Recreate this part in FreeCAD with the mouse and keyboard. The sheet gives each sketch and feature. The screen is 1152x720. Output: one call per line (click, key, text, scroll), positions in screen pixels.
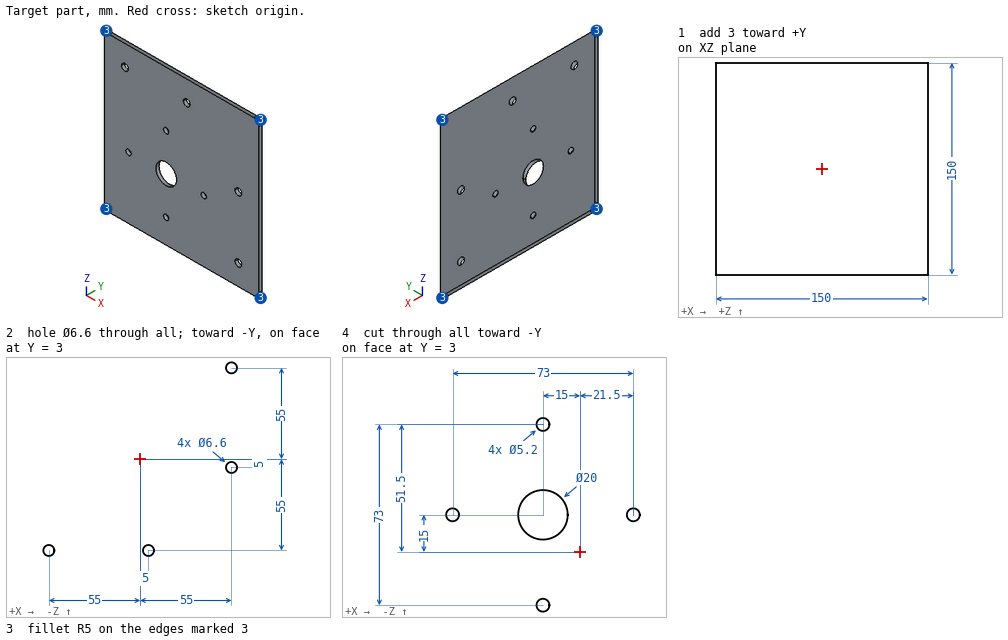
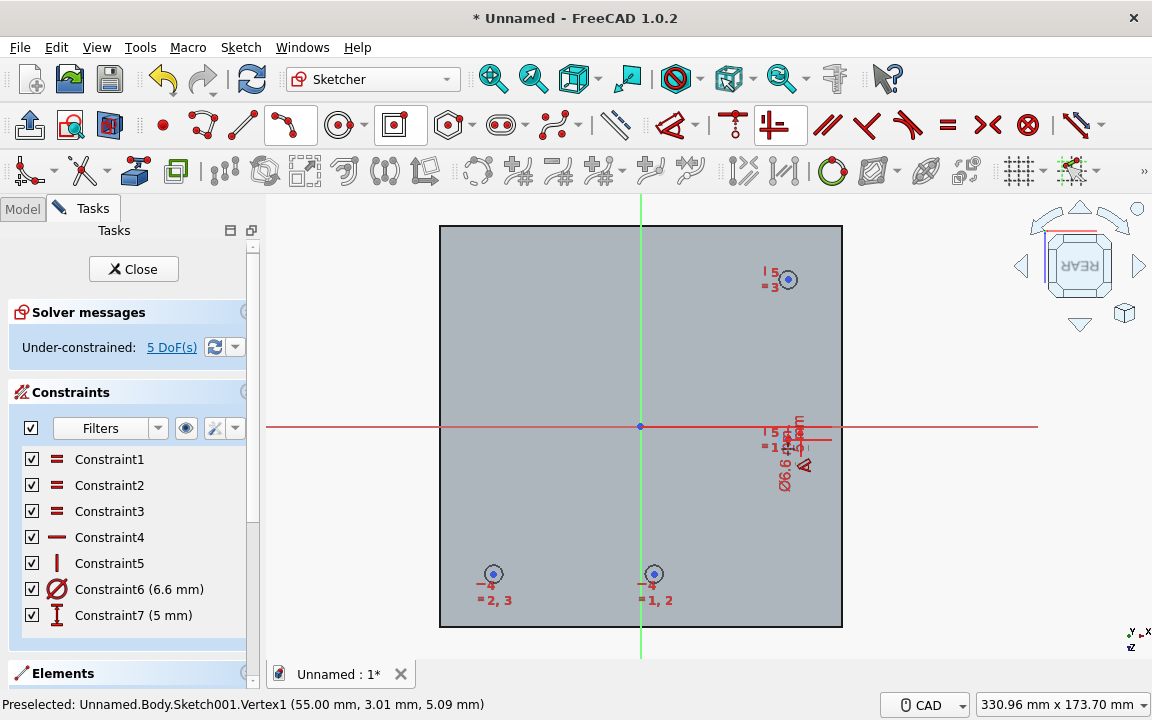
scroll(654, 574, up, 6)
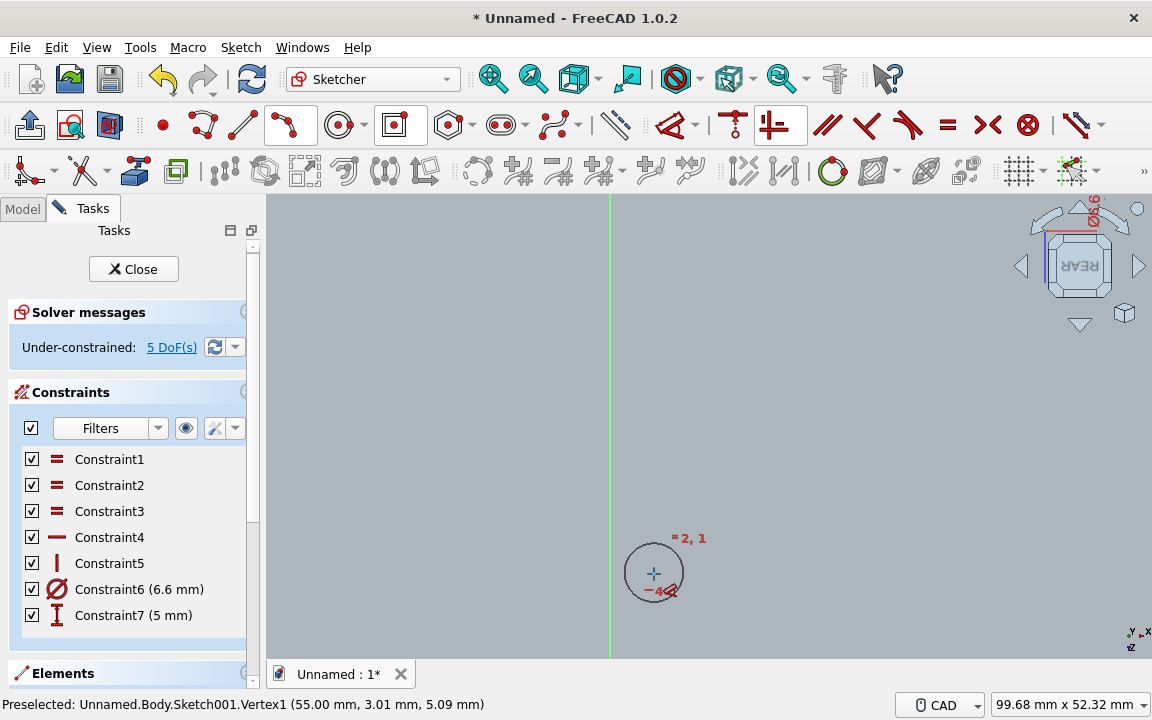
click(654, 573)
click(632, 631)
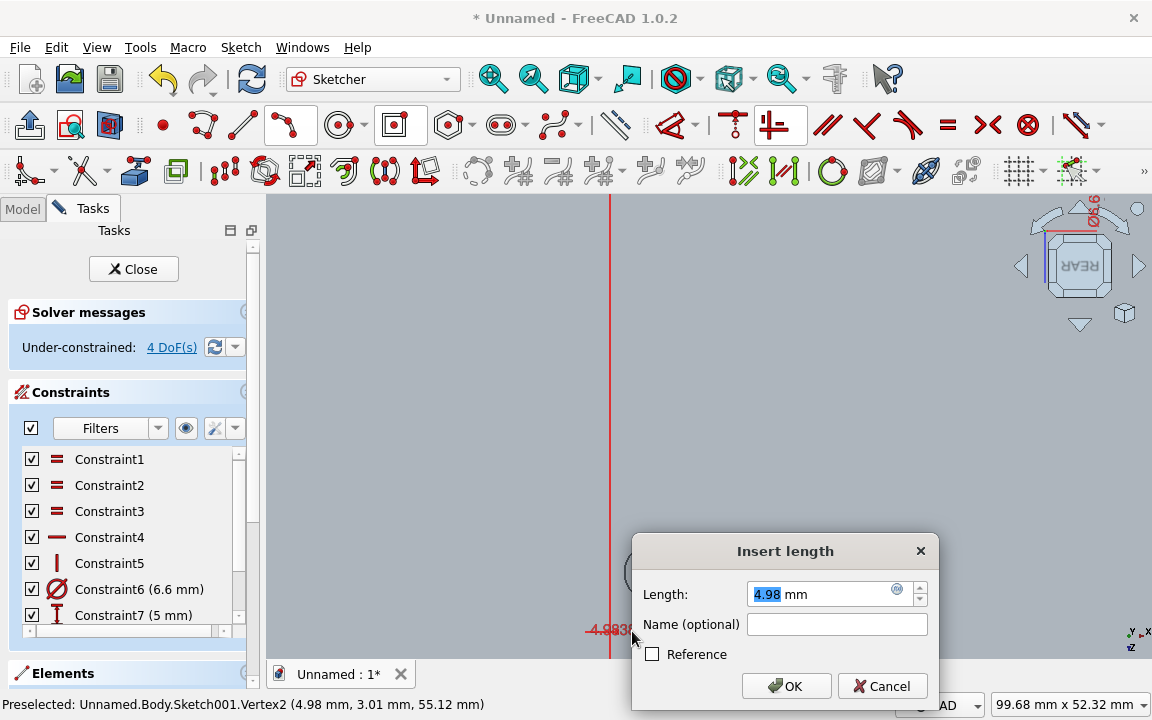
text(5)
key(Return)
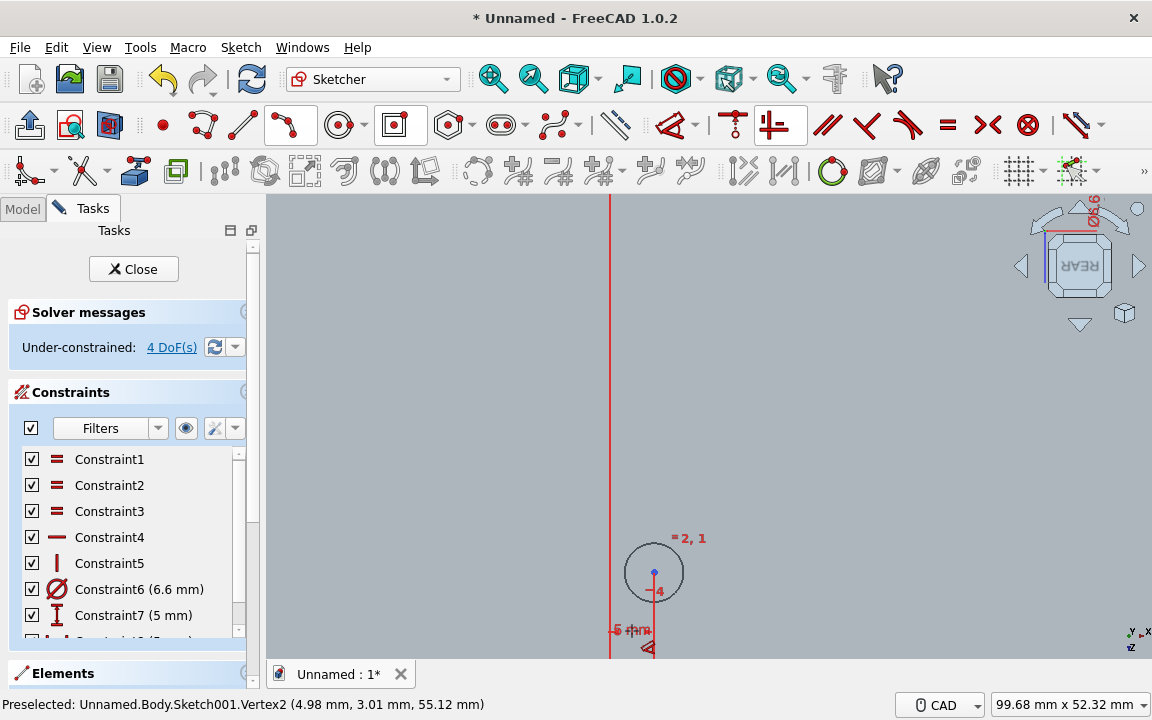
scroll(654, 575, down, 6)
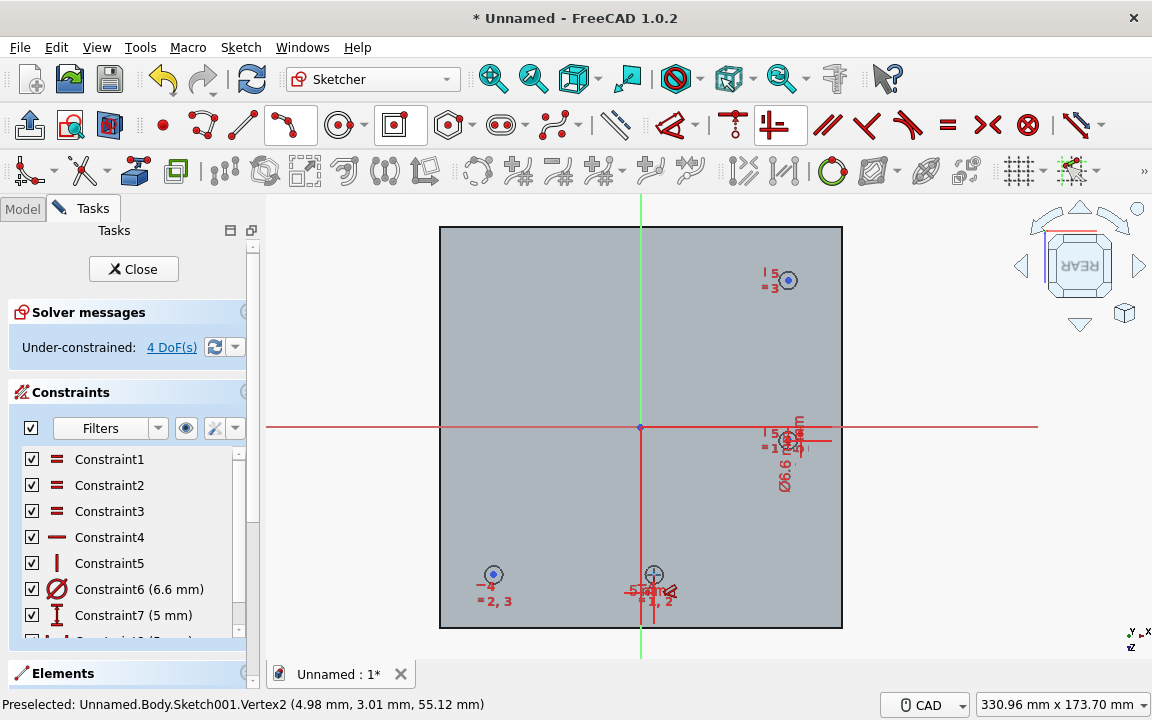
click(788, 441)
click(715, 475)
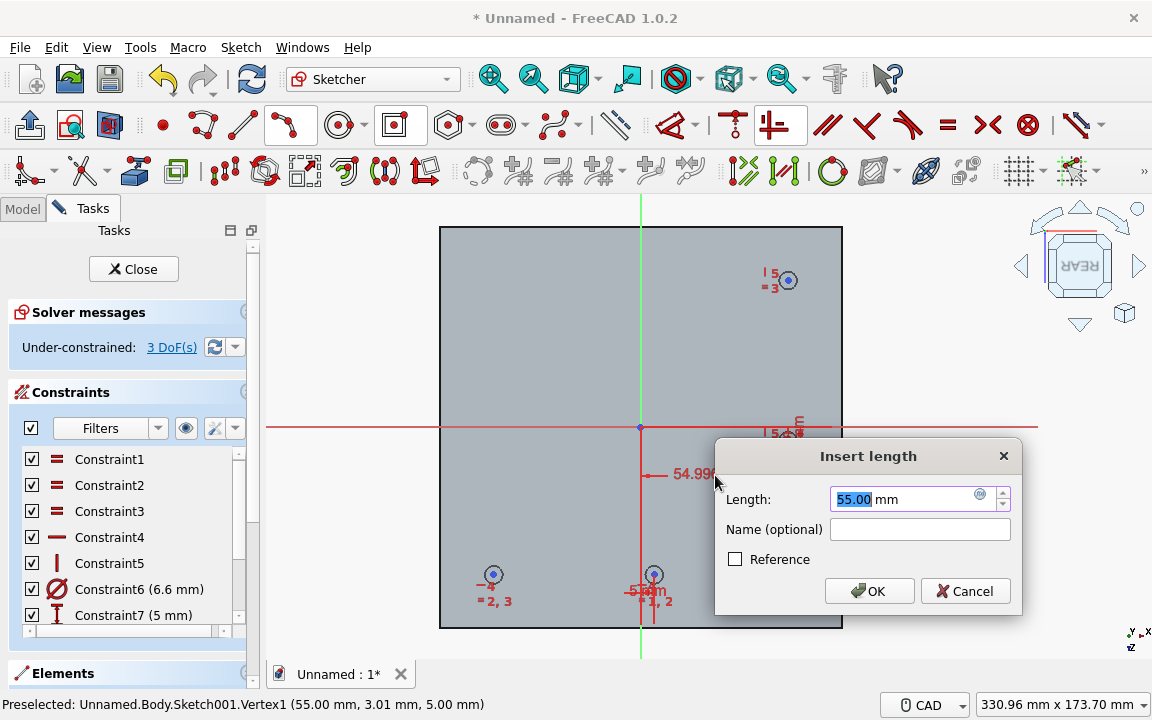
text(55)
key(Return)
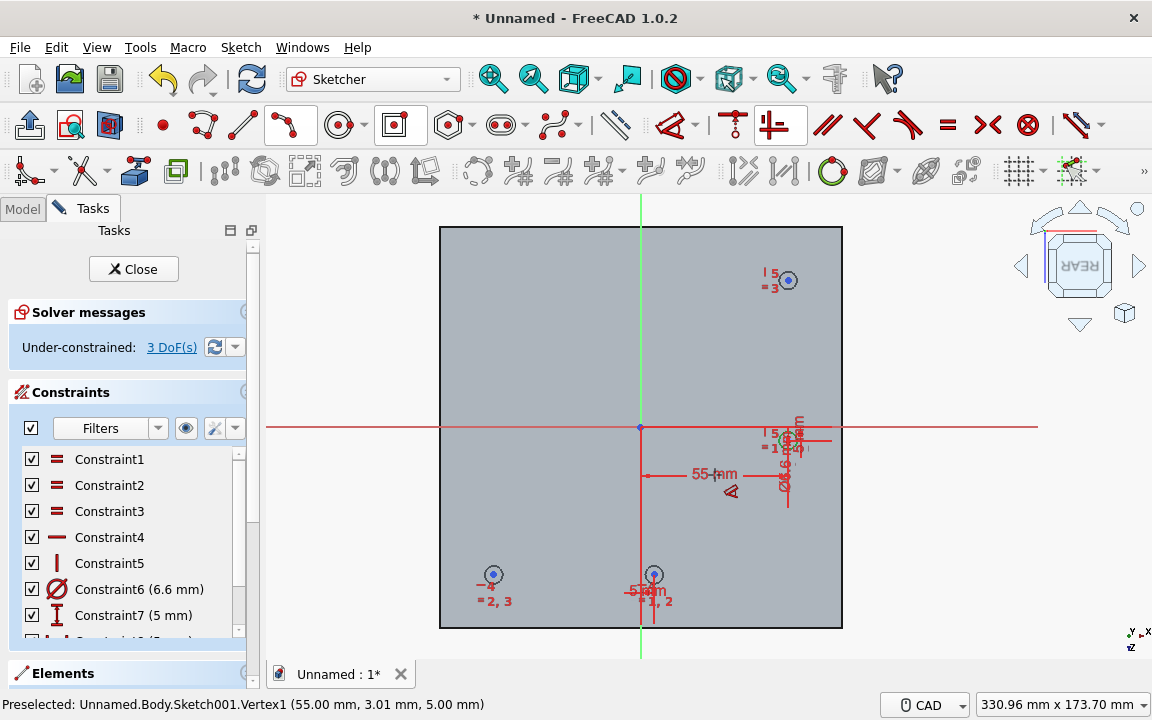
click(654, 575)
click(688, 501)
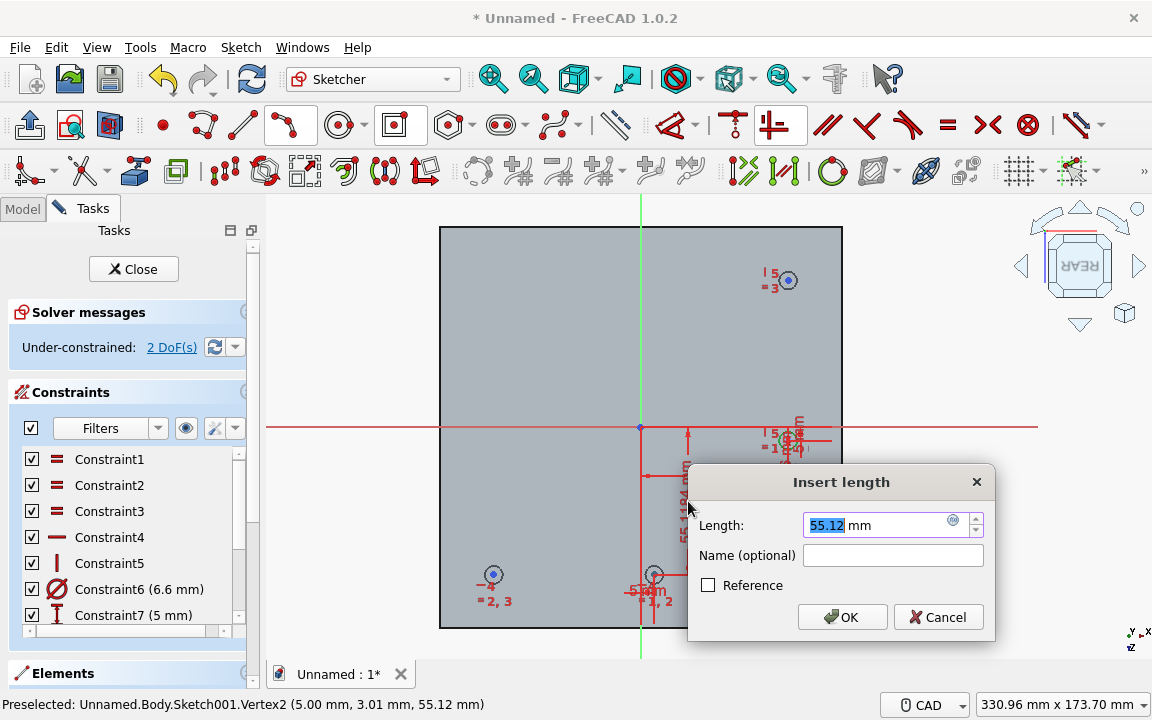
text(55)
key(Return)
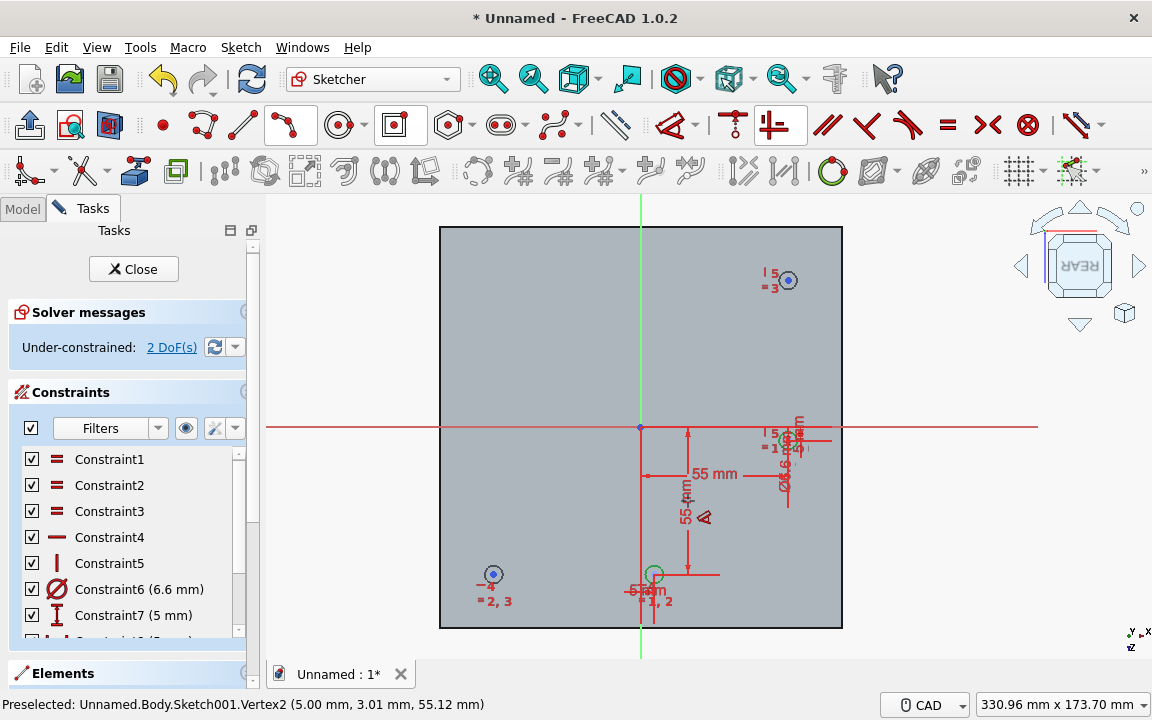
click(494, 575)
click(567, 609)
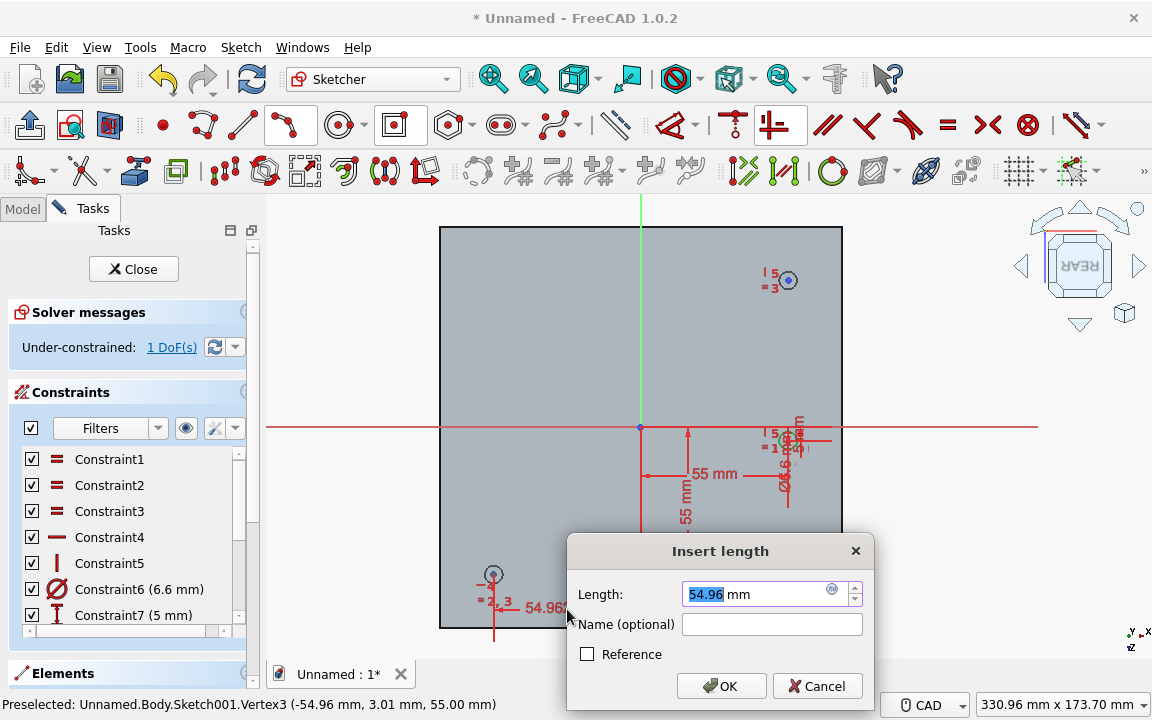
text(55)
key(Return)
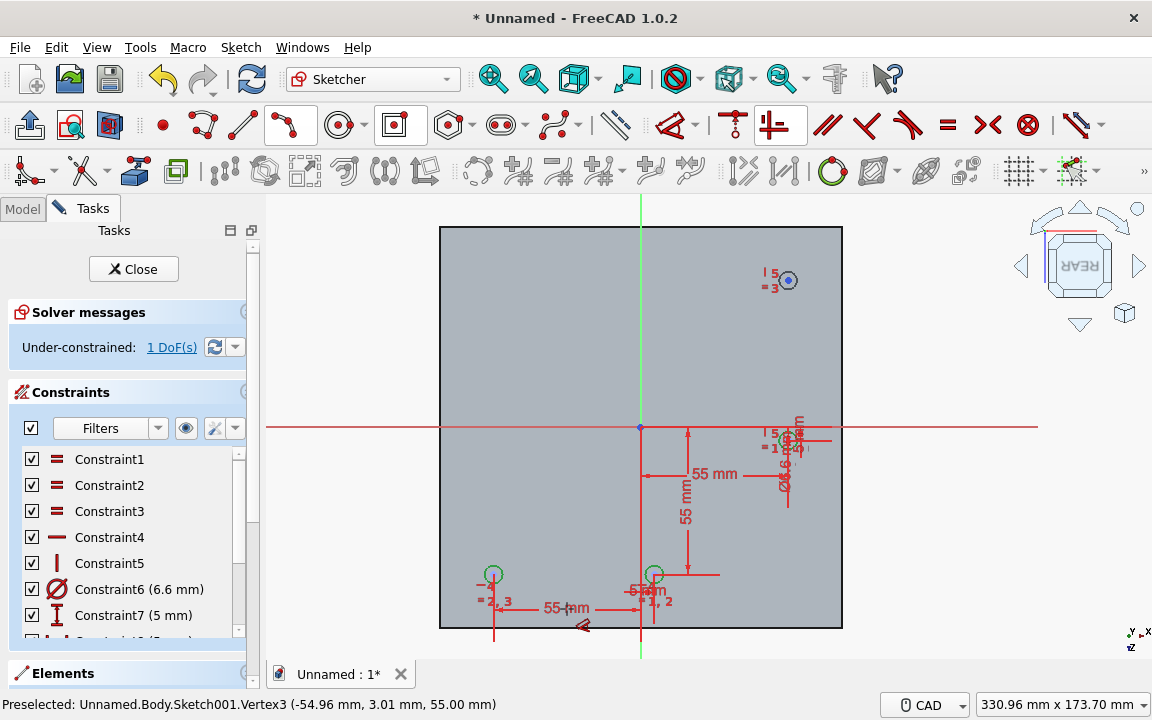
click(788, 281)
click(822, 354)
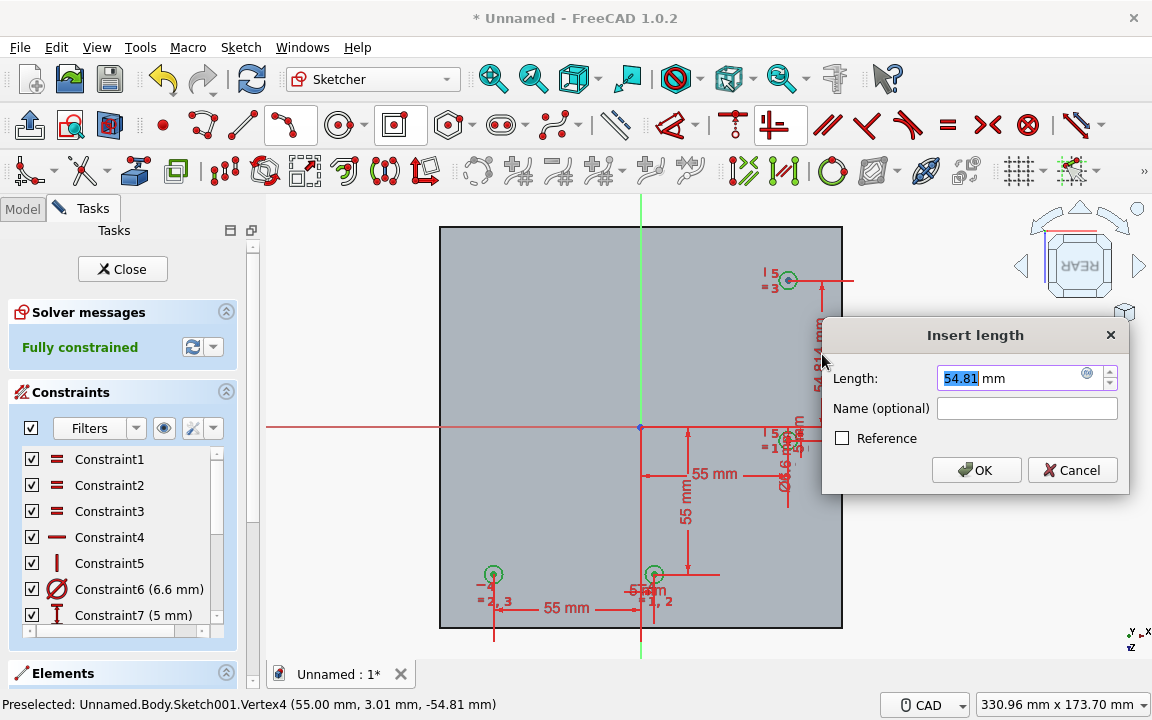
text(55)
key(Return)
key(Escape)